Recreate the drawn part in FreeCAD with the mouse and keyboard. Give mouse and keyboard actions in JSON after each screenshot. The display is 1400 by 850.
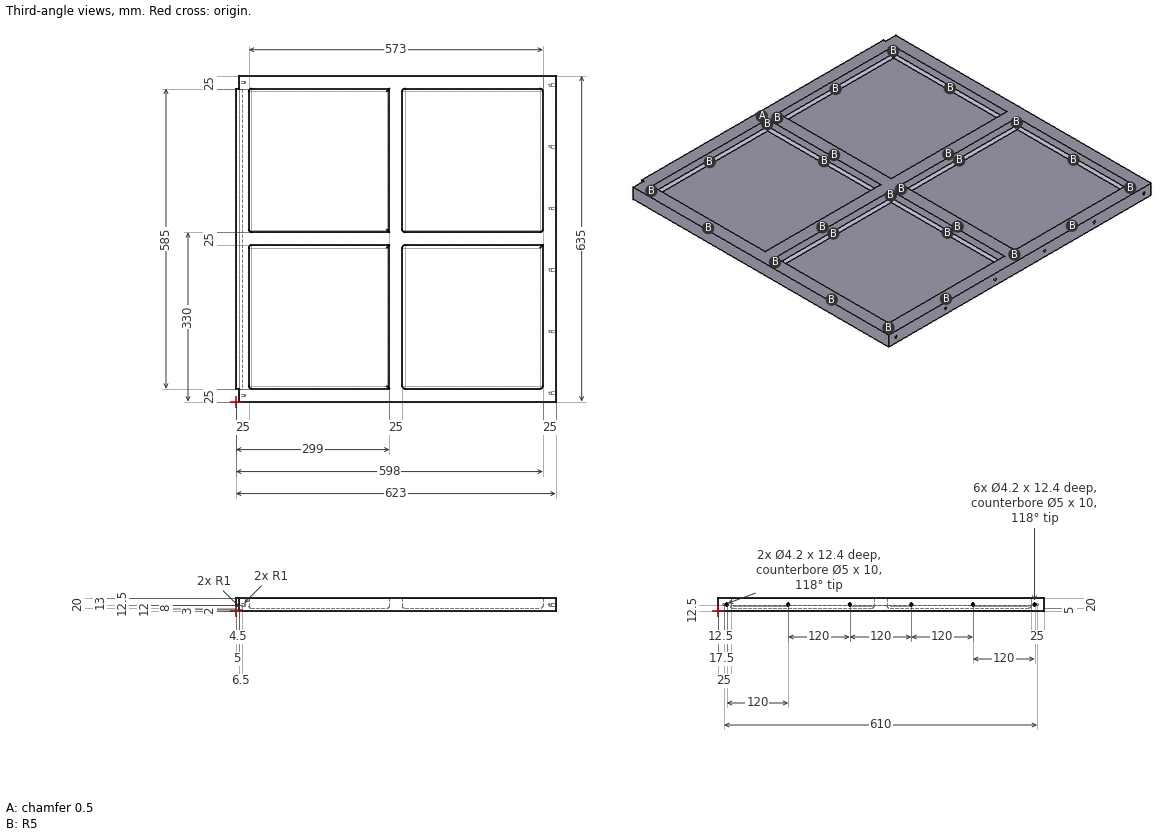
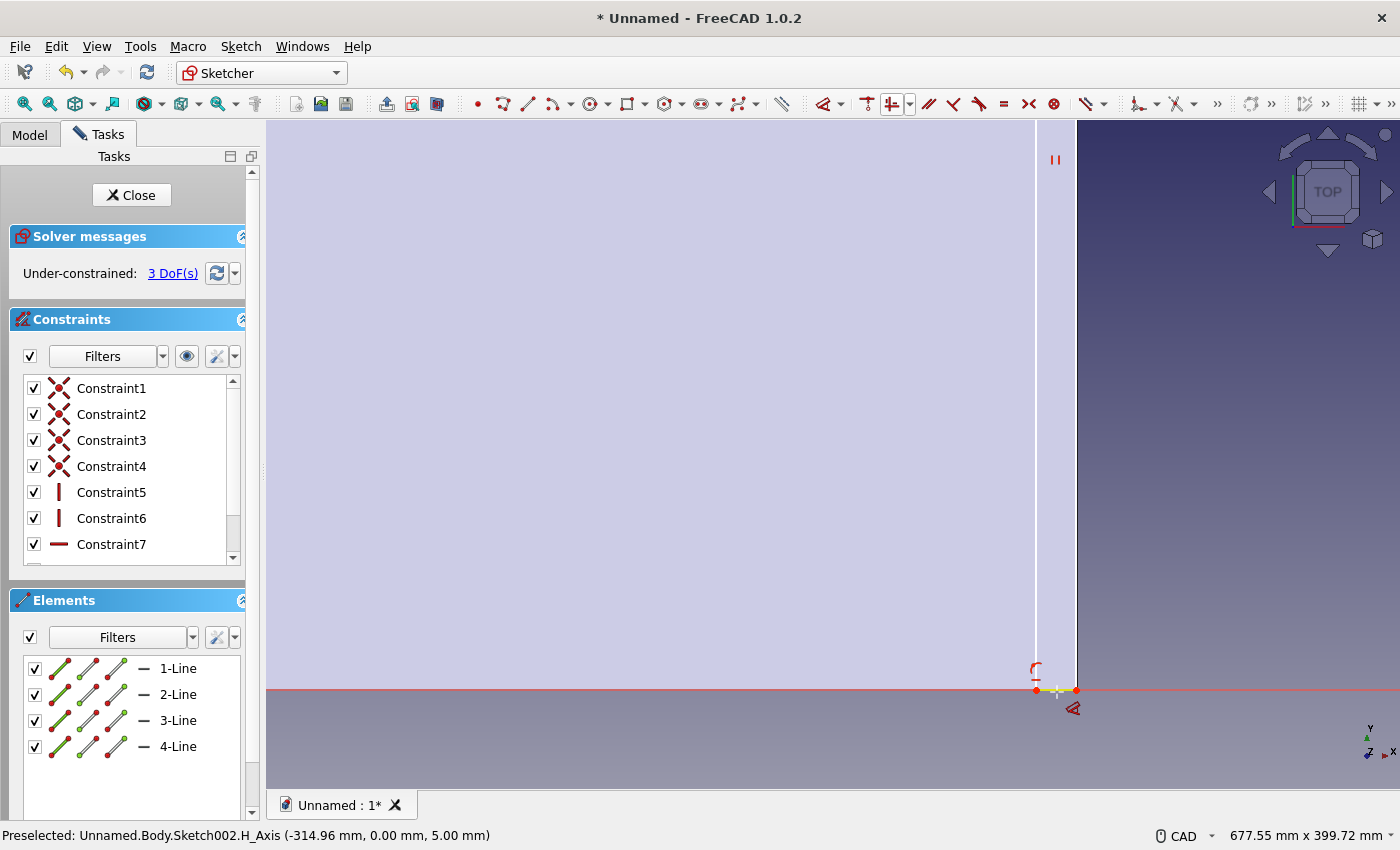
{"action": "left_click", "coordinate": [1056, 690]}
{"action": "left_click", "coordinate": [1056, 724]}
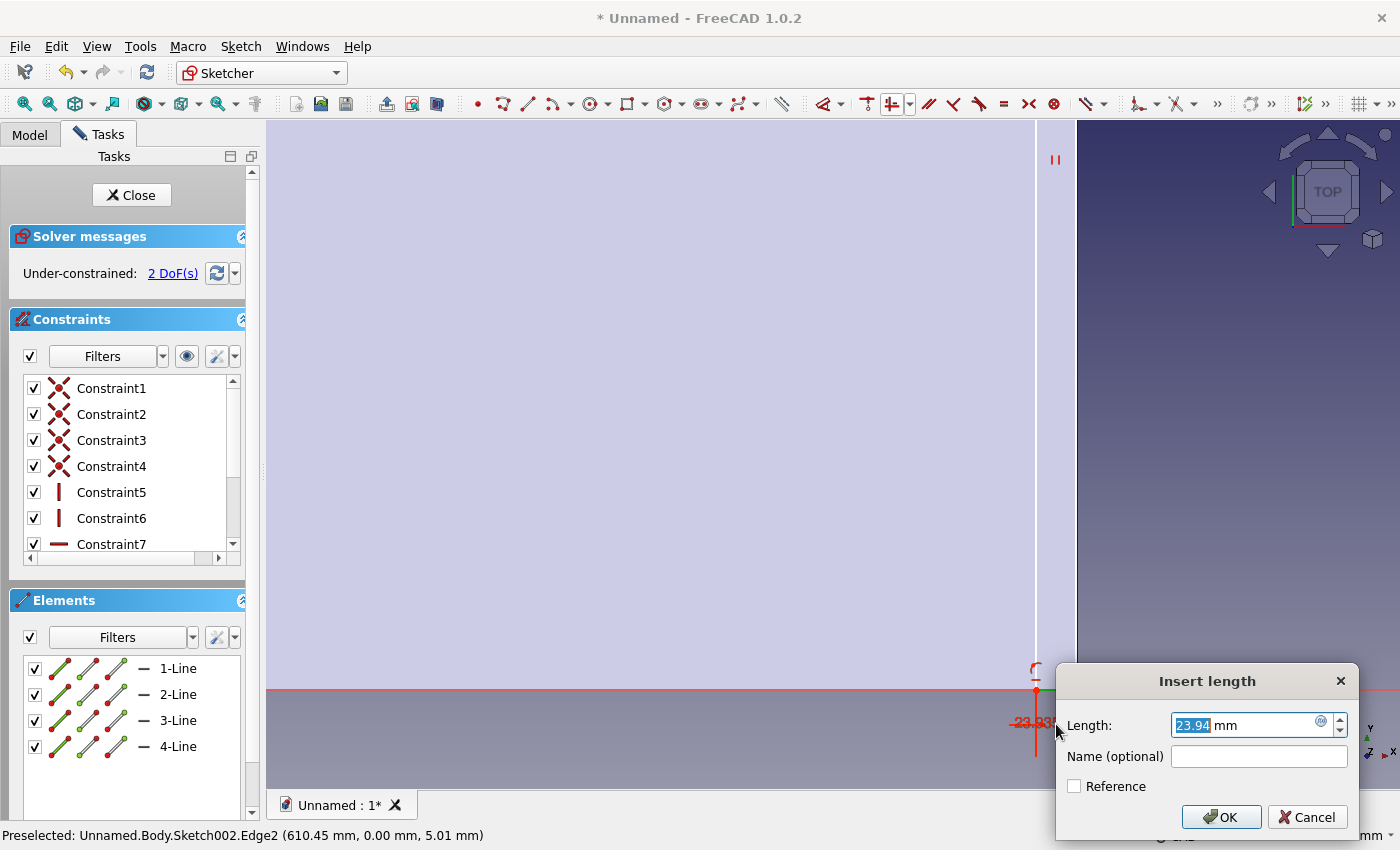
{"action": "type", "text": "25"}
{"action": "key", "text": "Return"}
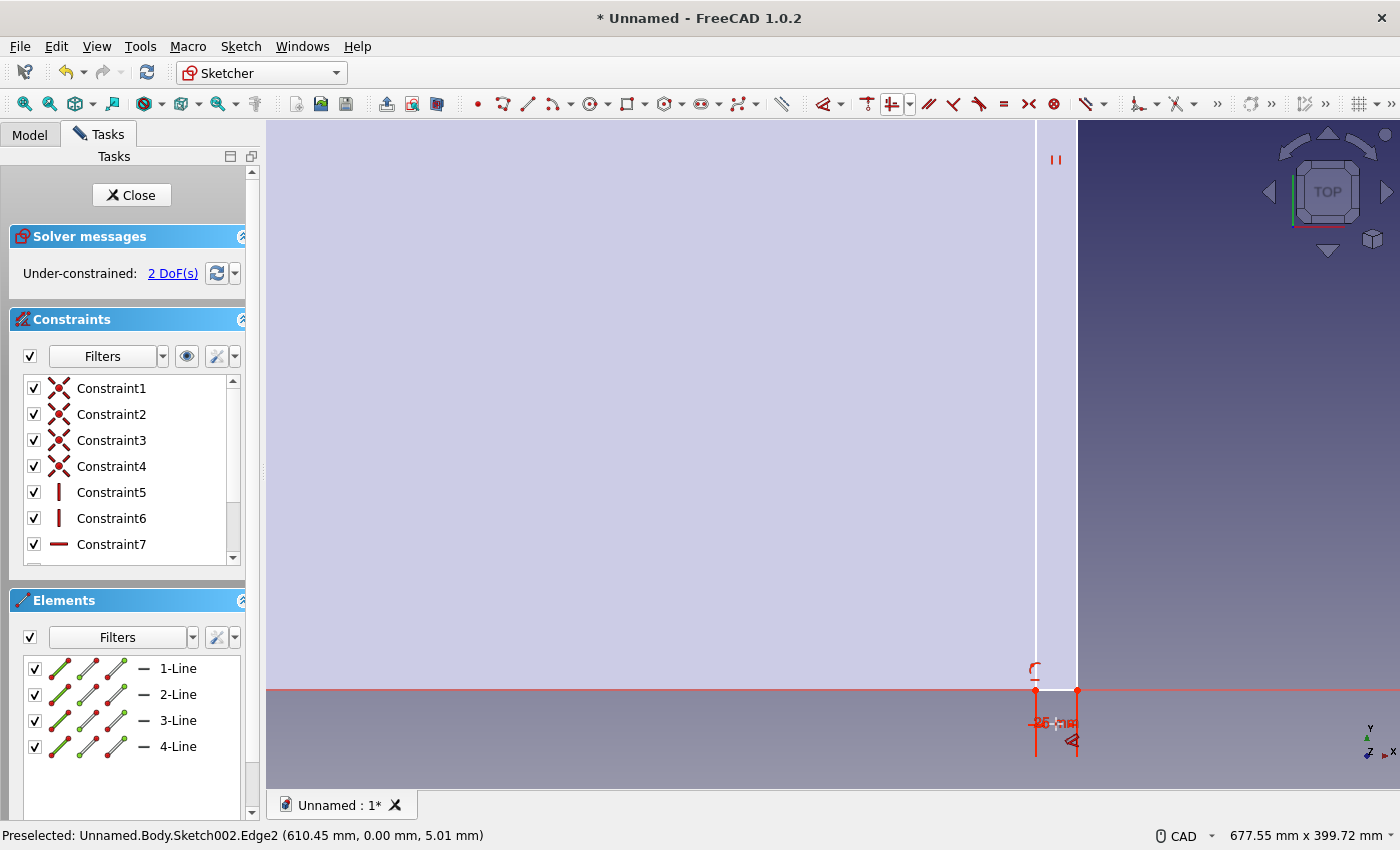
{"action": "left_click", "coordinate": [1036, 372]}
{"action": "left_click", "coordinate": [1002, 419]}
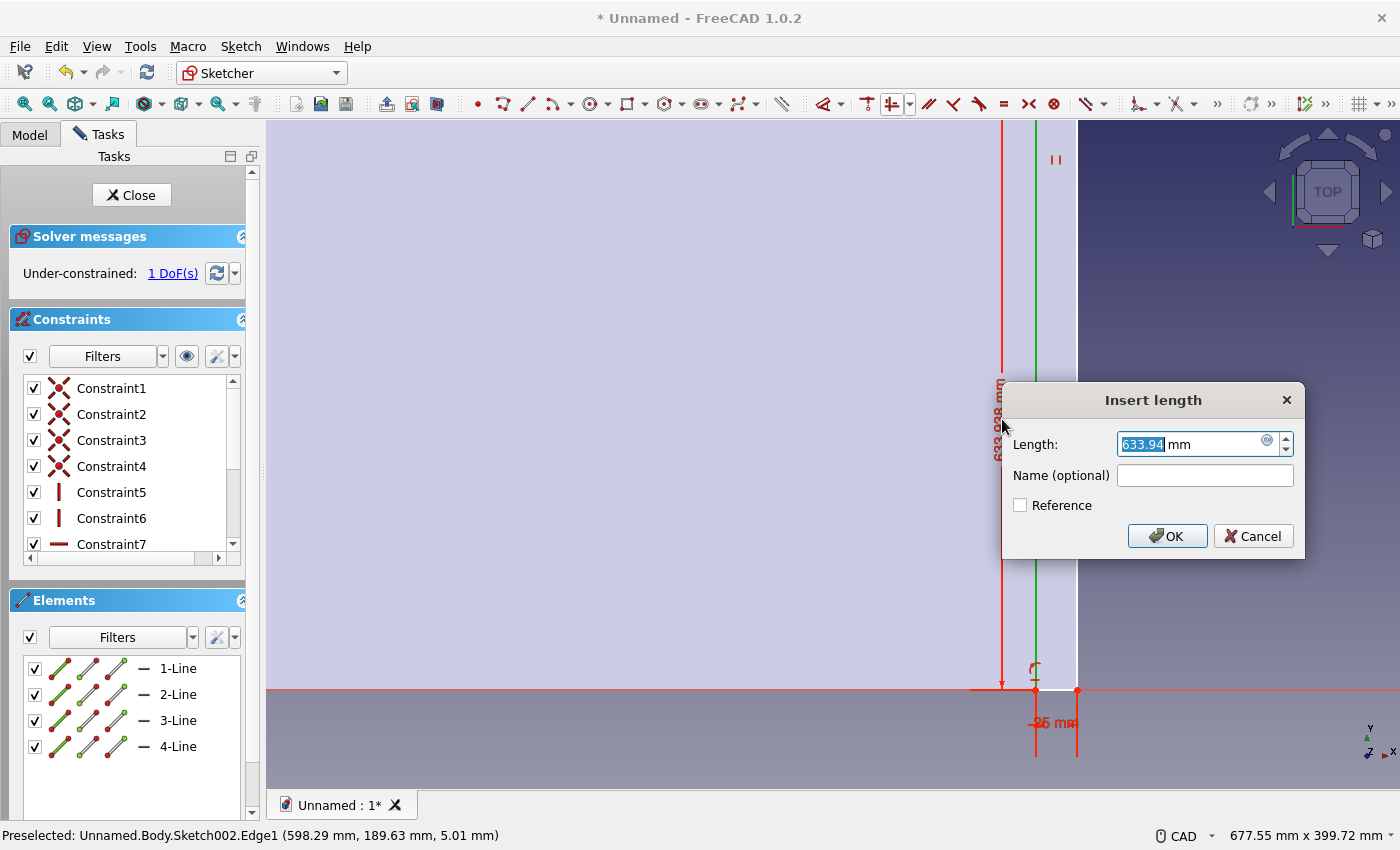
{"action": "type", "text": "635"}
{"action": "key", "text": "Return"}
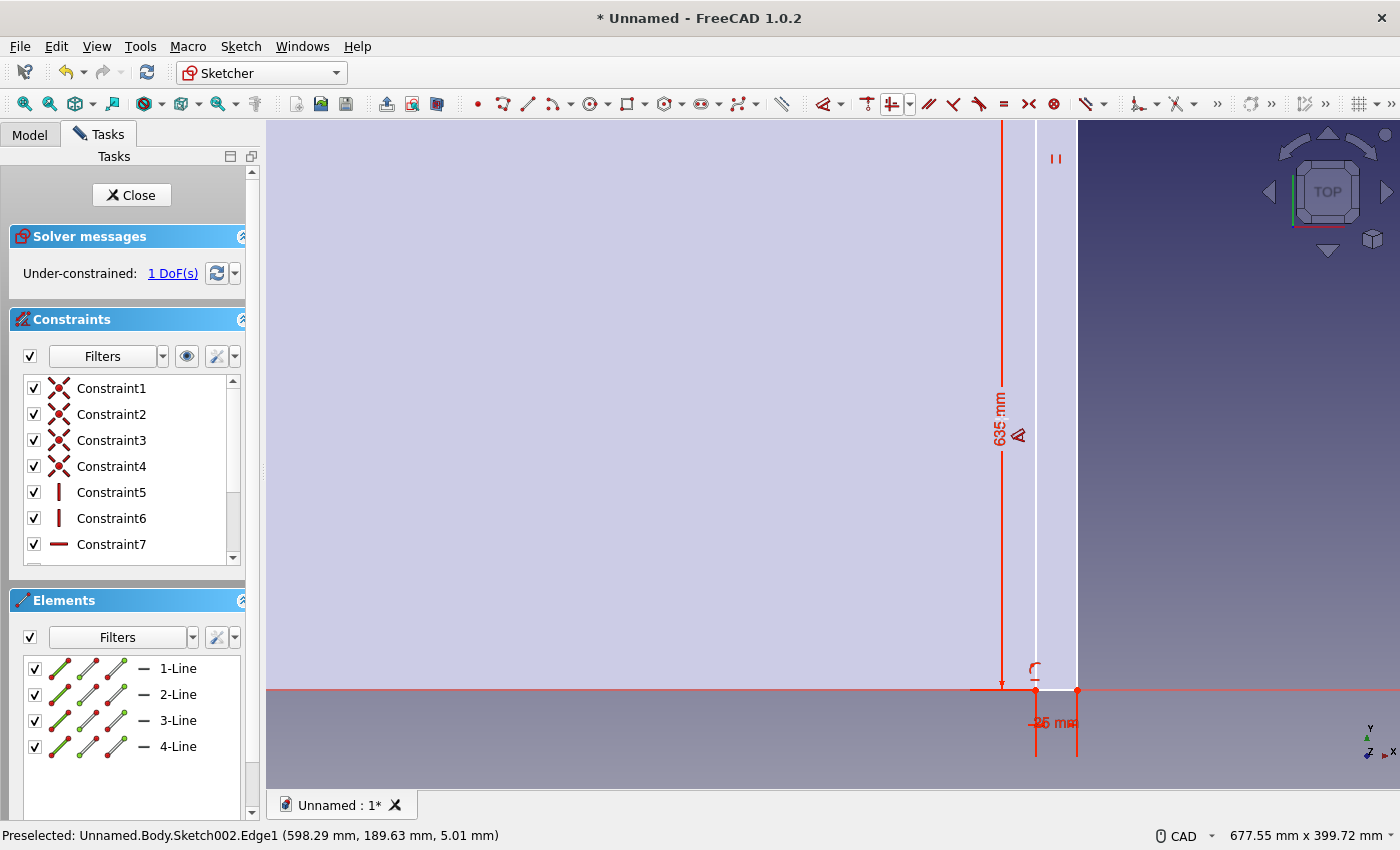
{"action": "scroll", "coordinate": [935, 696], "scroll_direction": "down", "scroll_amount": 4}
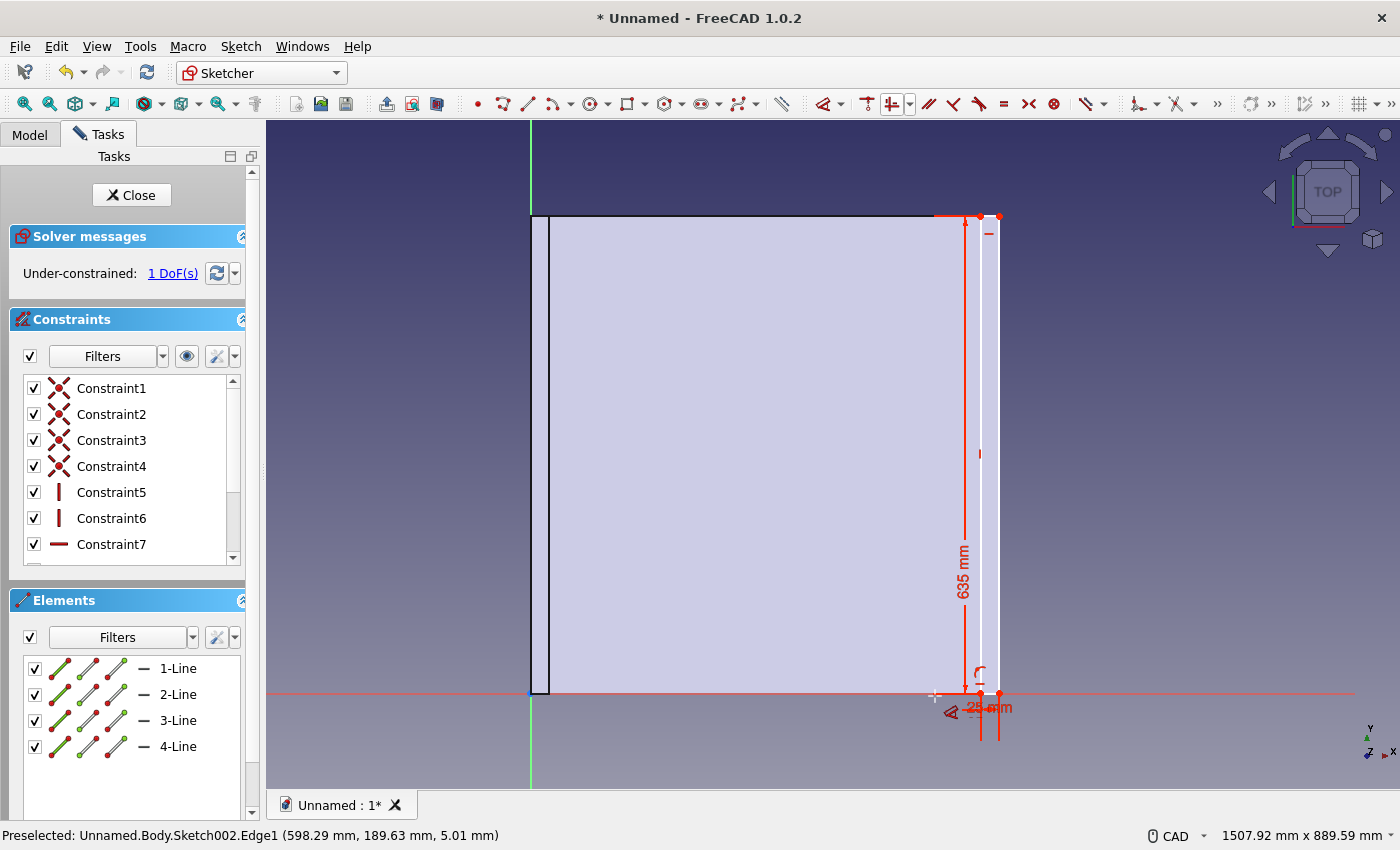
{"action": "left_click", "coordinate": [981, 216]}
{"action": "left_click", "coordinate": [756, 728]}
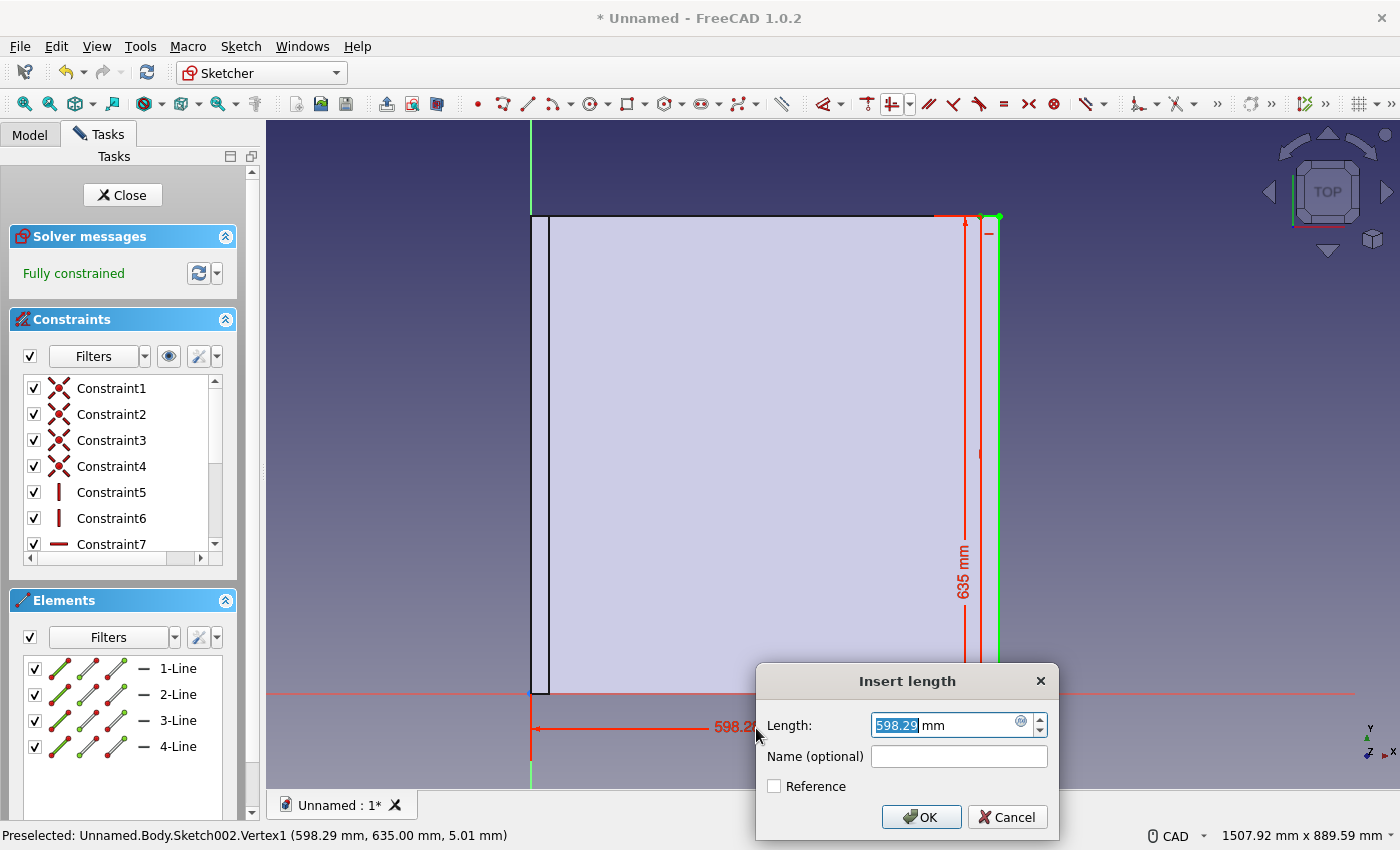
{"action": "type", "text": "598"}
{"action": "key", "text": "Return"}
{"action": "key", "text": "Escape"}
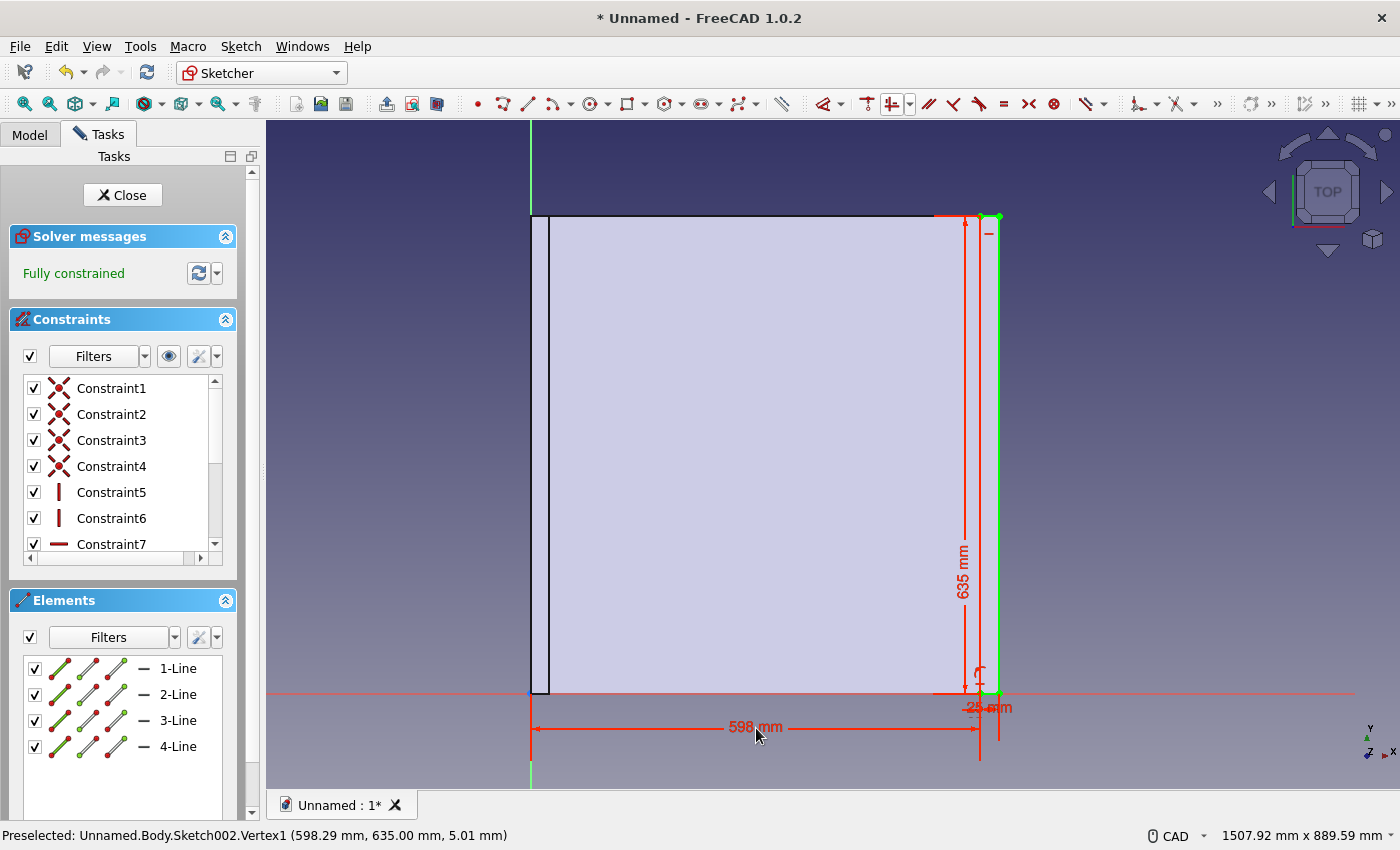
{"action": "left_click", "coordinate": [123, 195]}